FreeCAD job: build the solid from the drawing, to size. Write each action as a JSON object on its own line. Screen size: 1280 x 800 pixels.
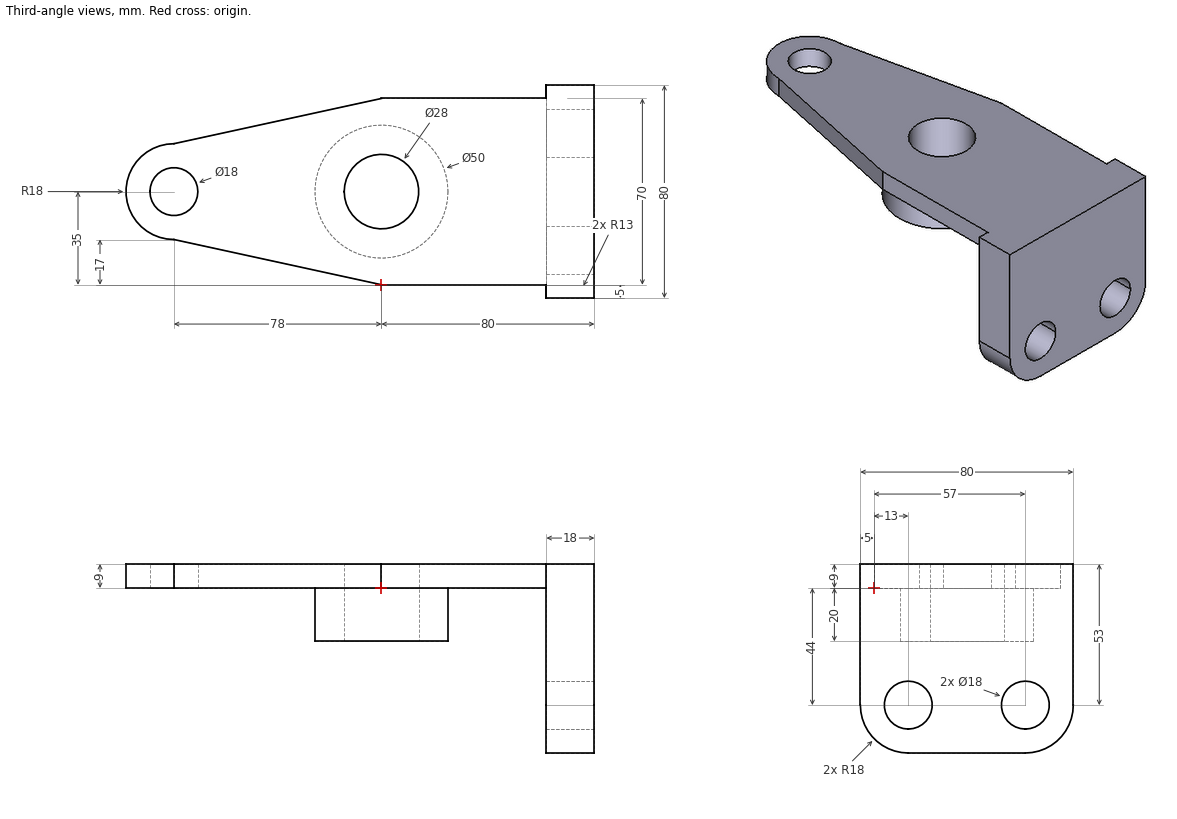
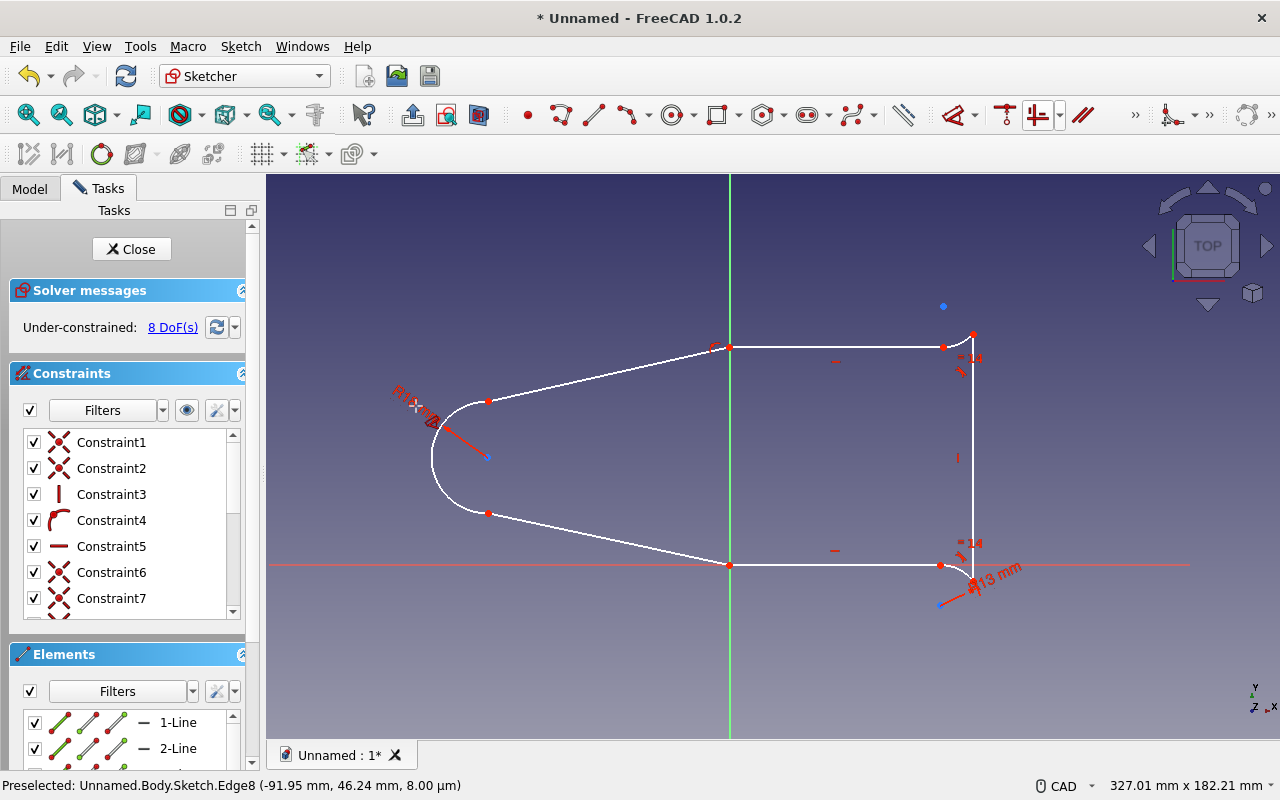
{"action": "left_click", "coordinate": [973, 507]}
{"action": "left_click", "coordinate": [1007, 458]}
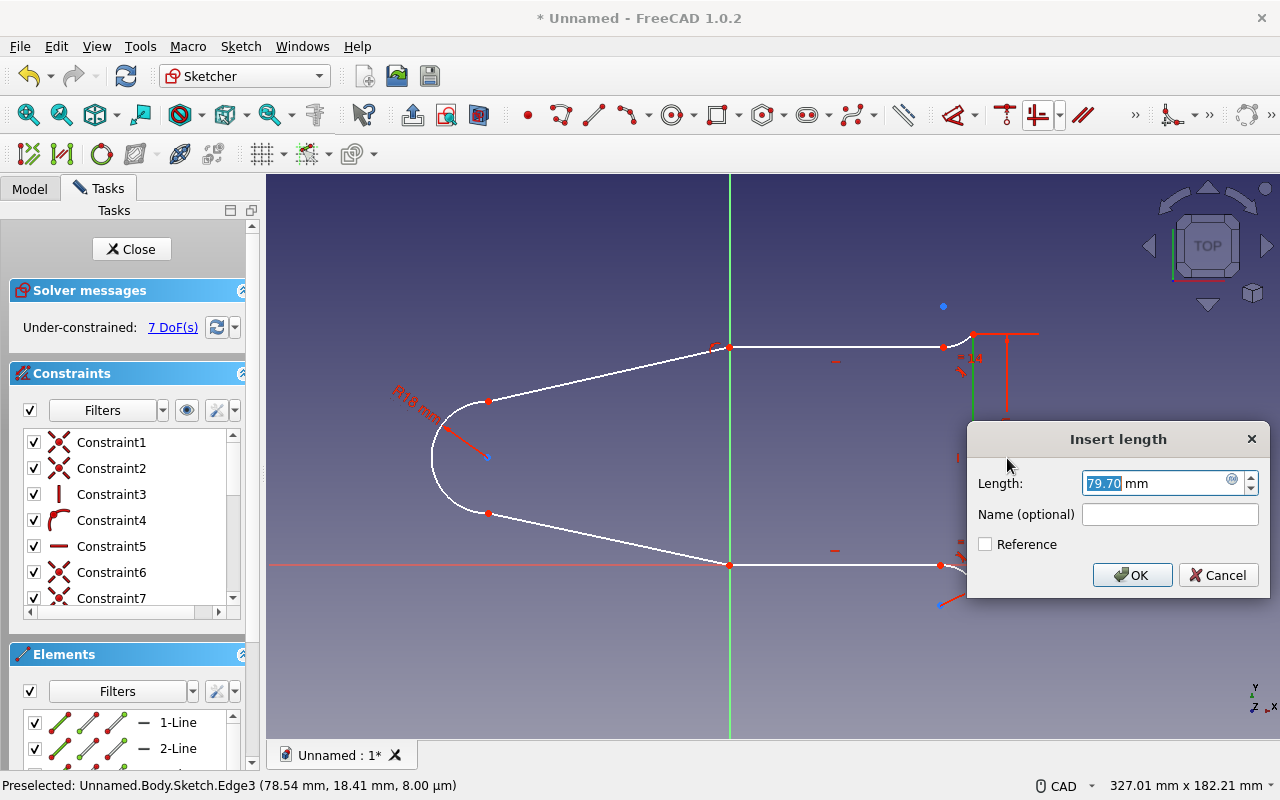
{"action": "type", "text": "80"}
{"action": "key", "text": "Return"}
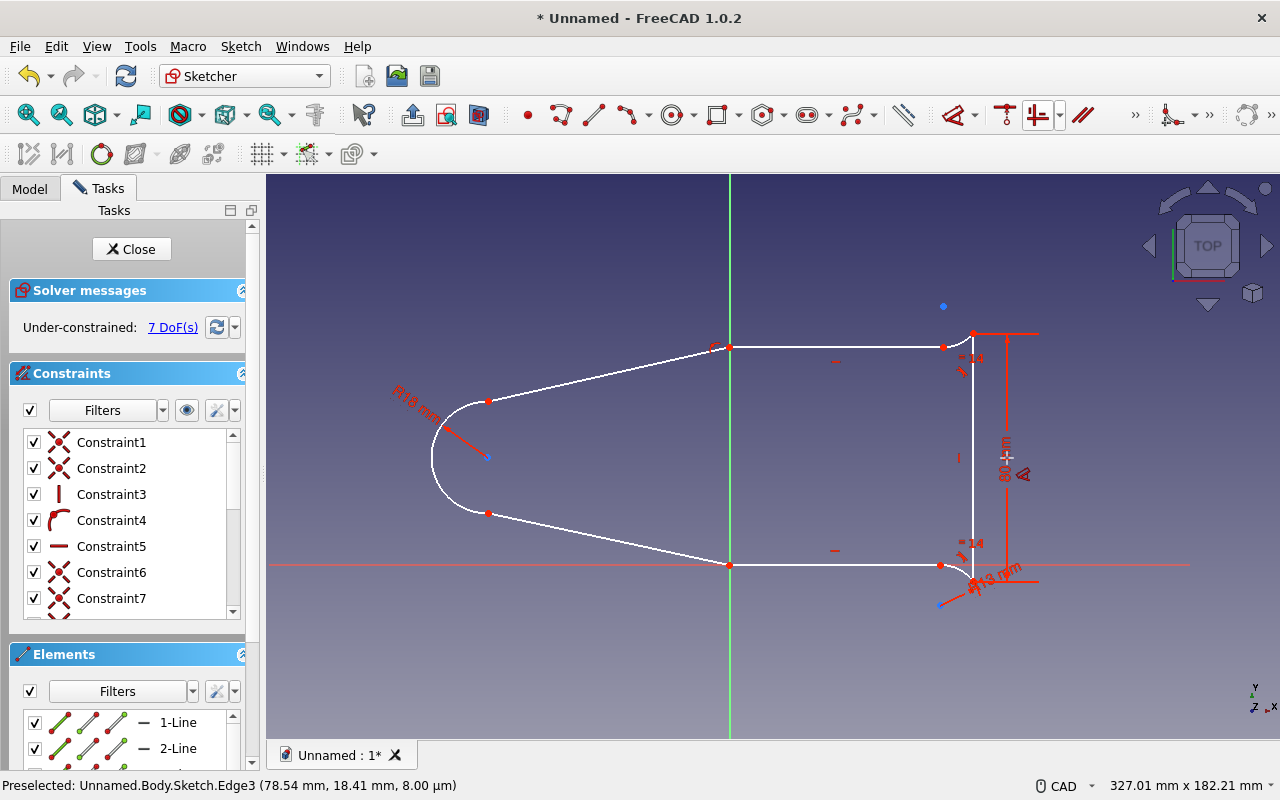
{"action": "scroll", "coordinate": [973, 582], "scroll_direction": "up", "scroll_amount": 5}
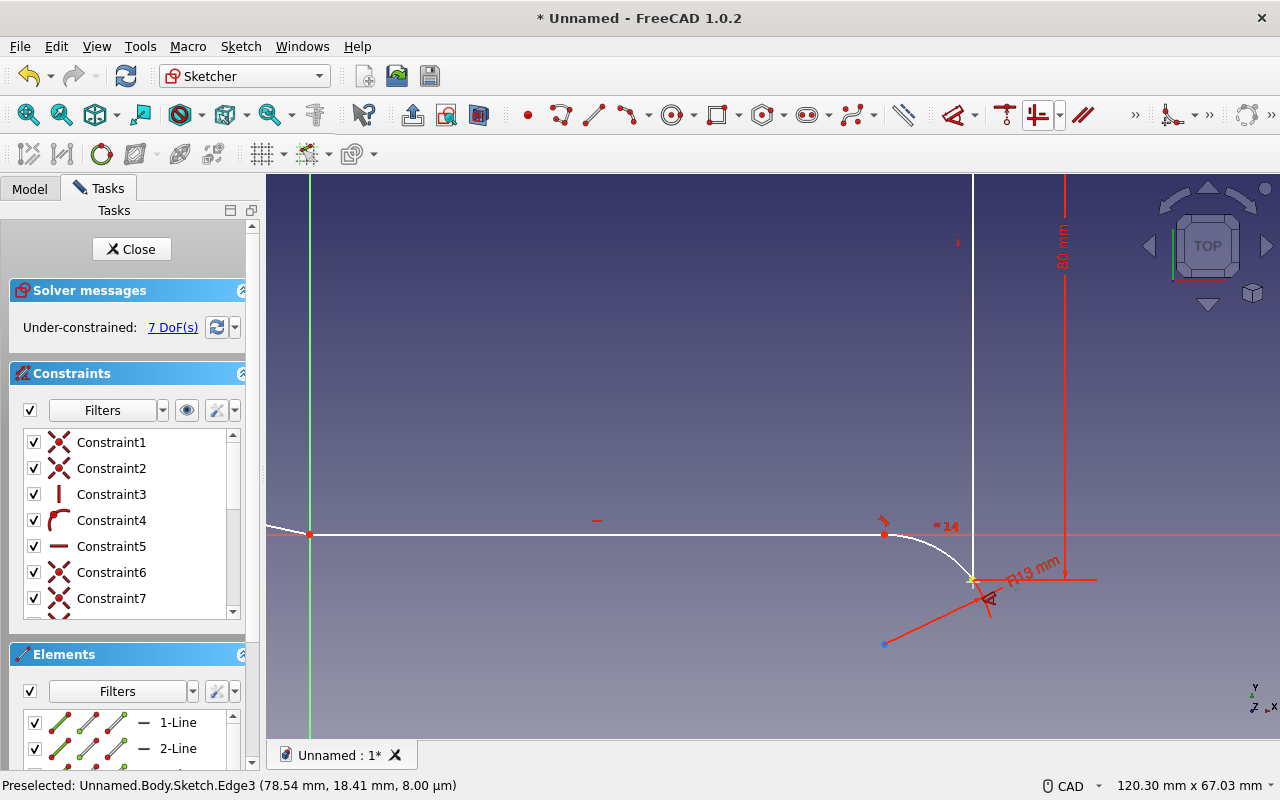
{"action": "left_click", "coordinate": [973, 580]}
{"action": "left_click", "coordinate": [1007, 557]}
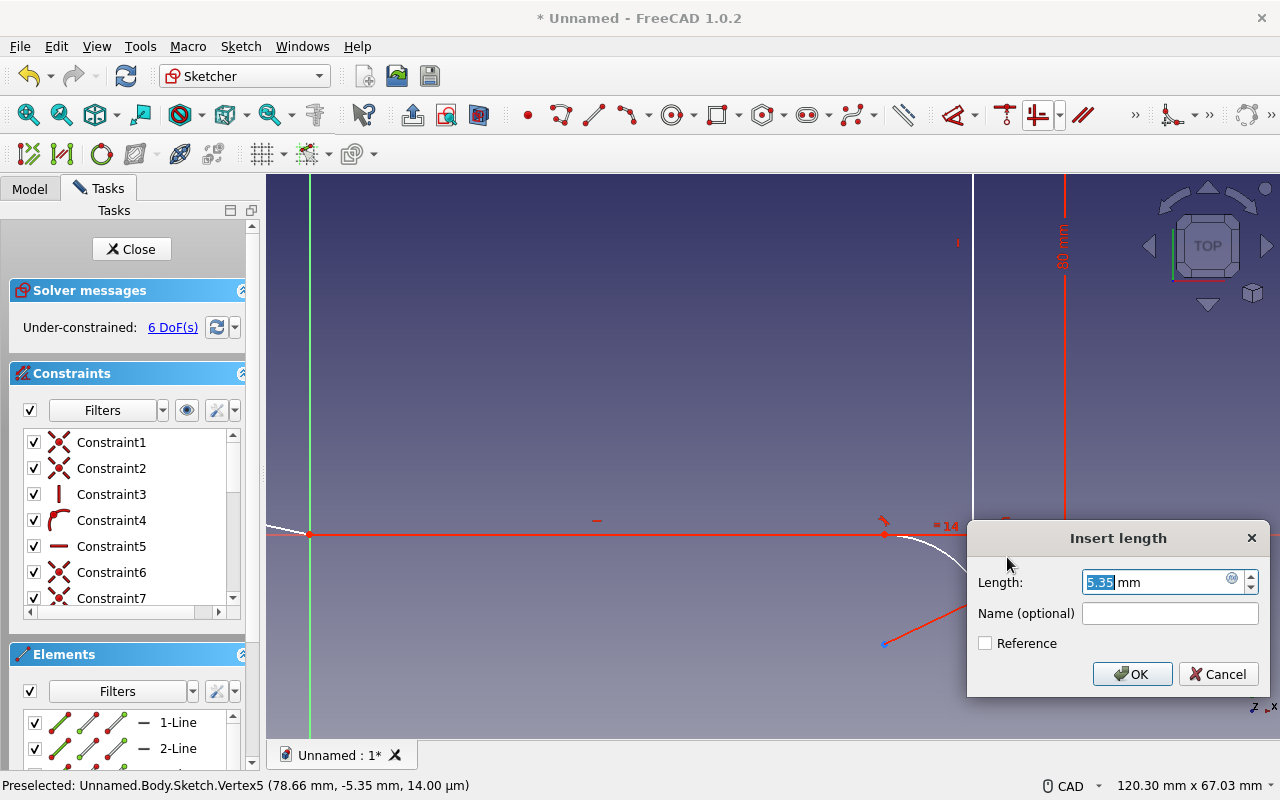
{"action": "type", "text": "5"}
{"action": "key", "text": "Return"}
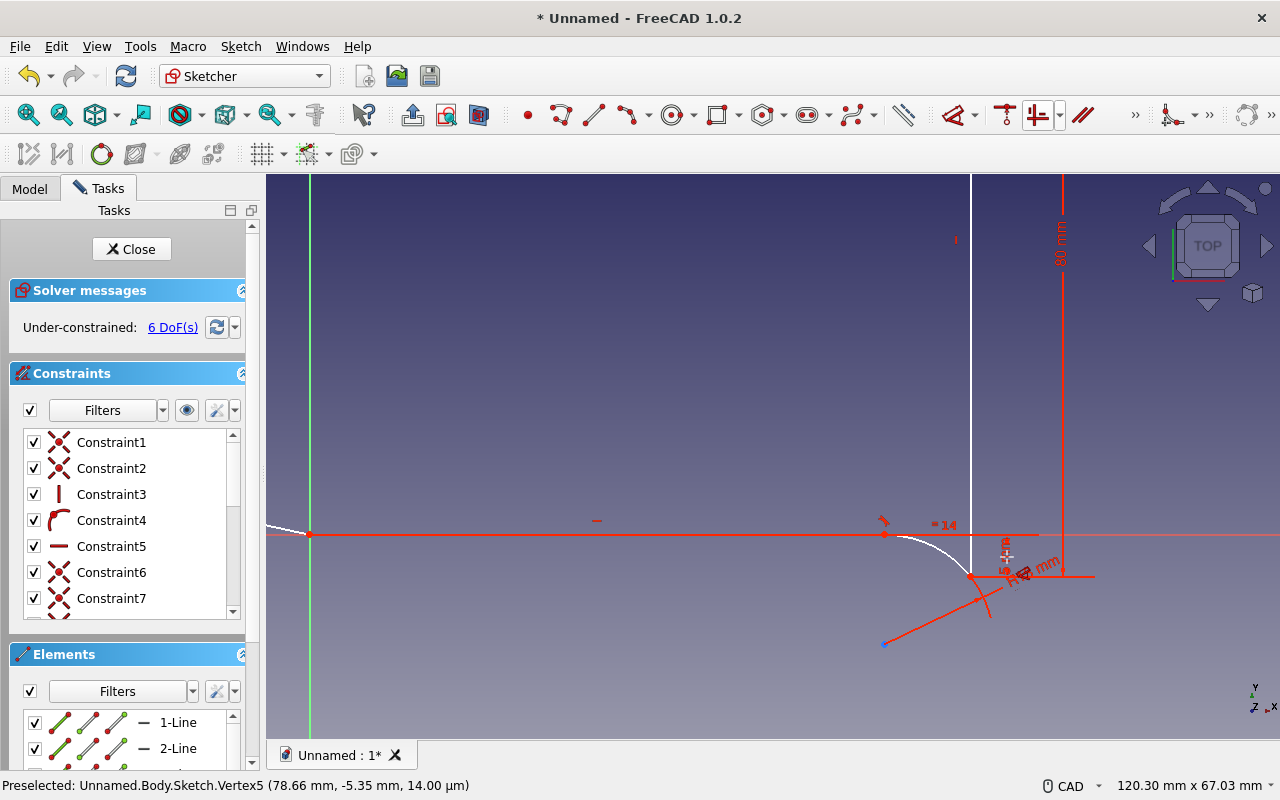
{"action": "scroll", "coordinate": [973, 583], "scroll_direction": "down", "scroll_amount": 5}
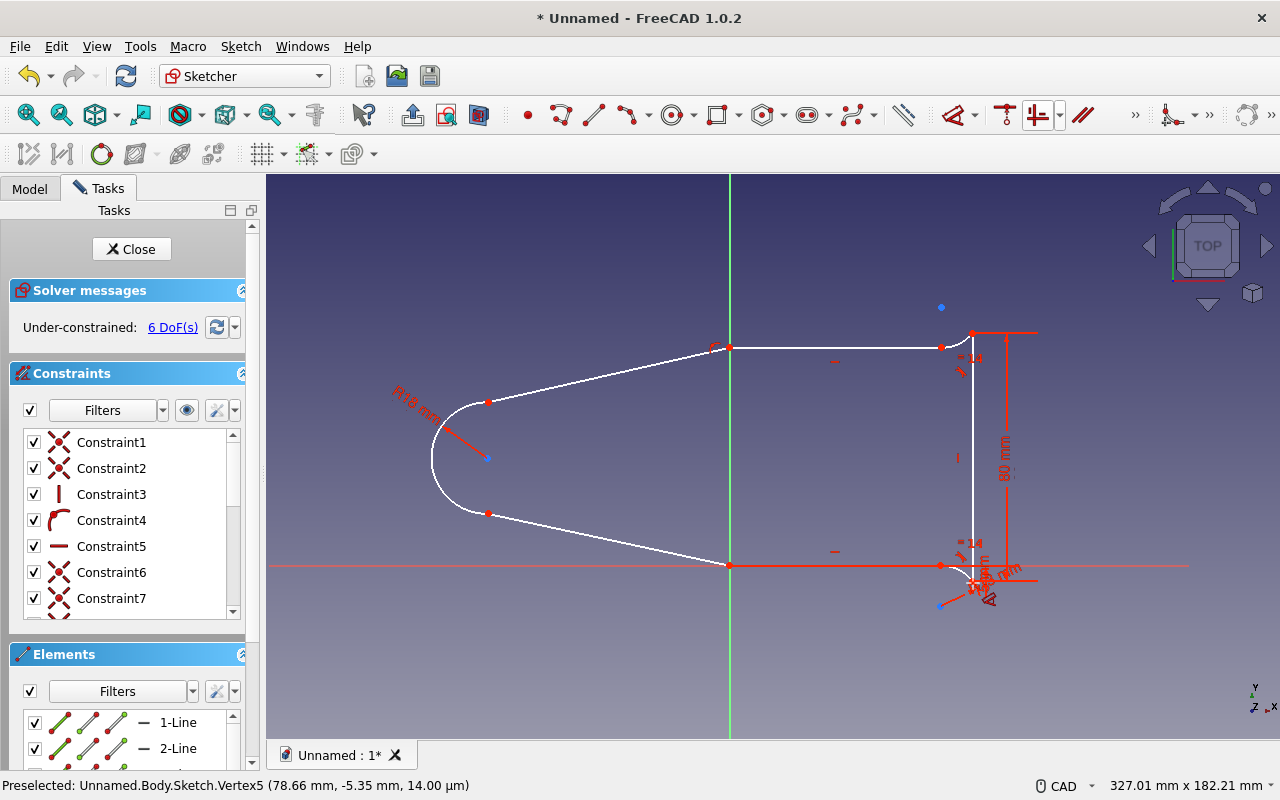
{"action": "left_click", "coordinate": [488, 514]}
{"action": "left_click", "coordinate": [609, 600]}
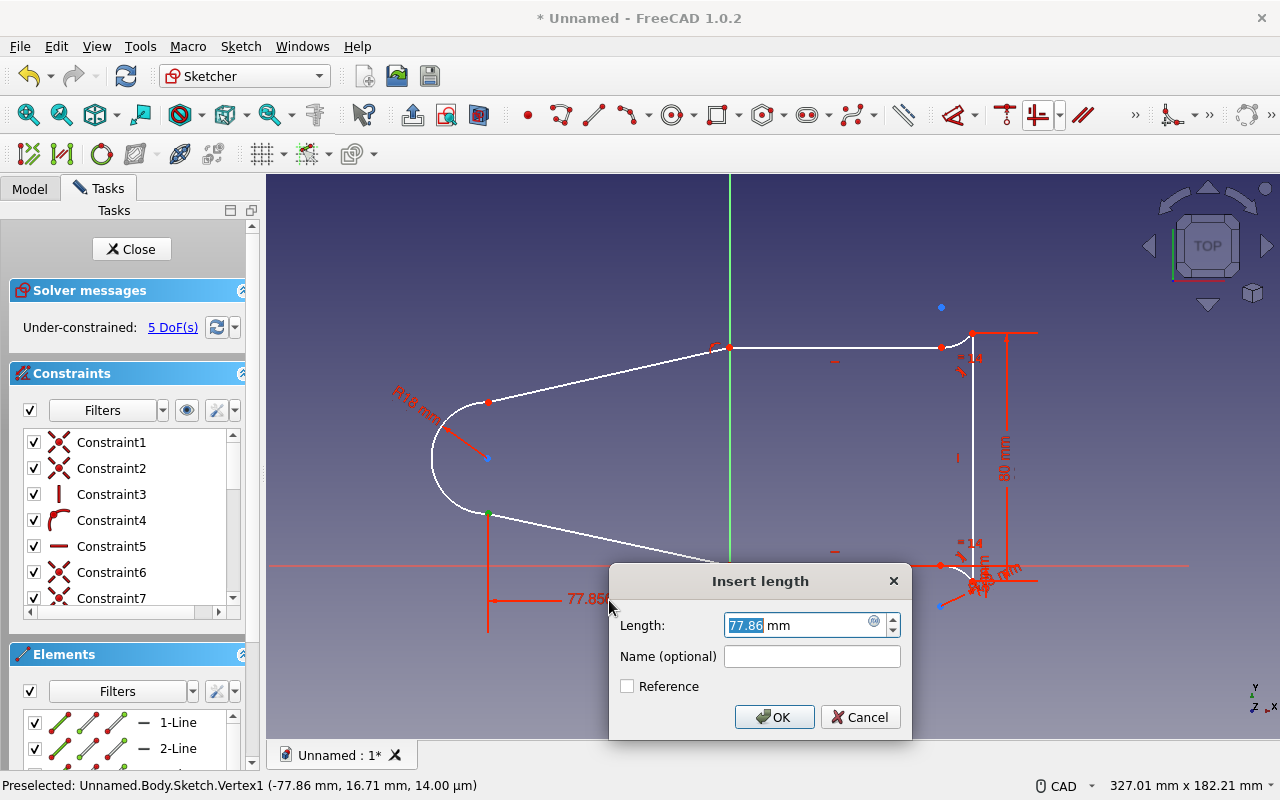
{"action": "type", "text": "78"}
{"action": "key", "text": "Return"}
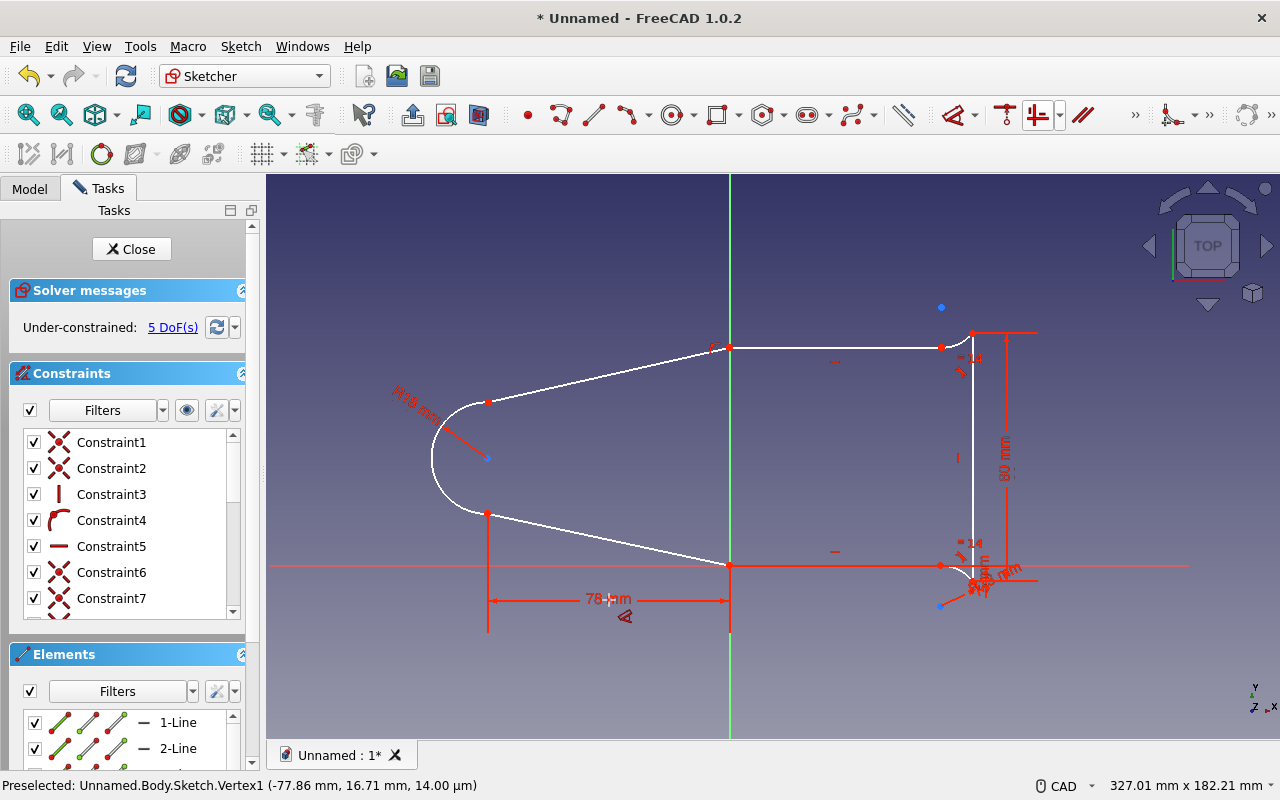
{"action": "left_click", "coordinate": [488, 514]}
{"action": "left_click", "coordinate": [454, 540]}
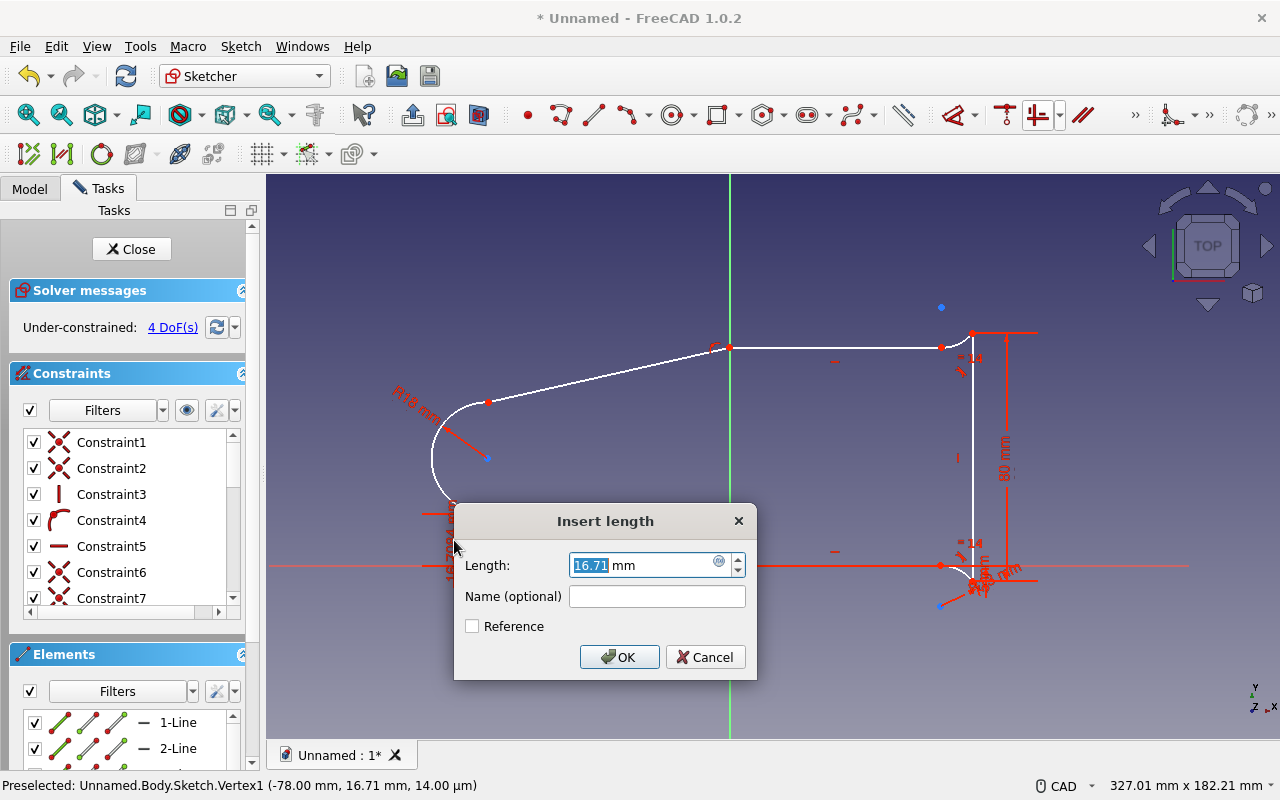
{"action": "type", "text": "17"}
{"action": "key", "text": "Return"}